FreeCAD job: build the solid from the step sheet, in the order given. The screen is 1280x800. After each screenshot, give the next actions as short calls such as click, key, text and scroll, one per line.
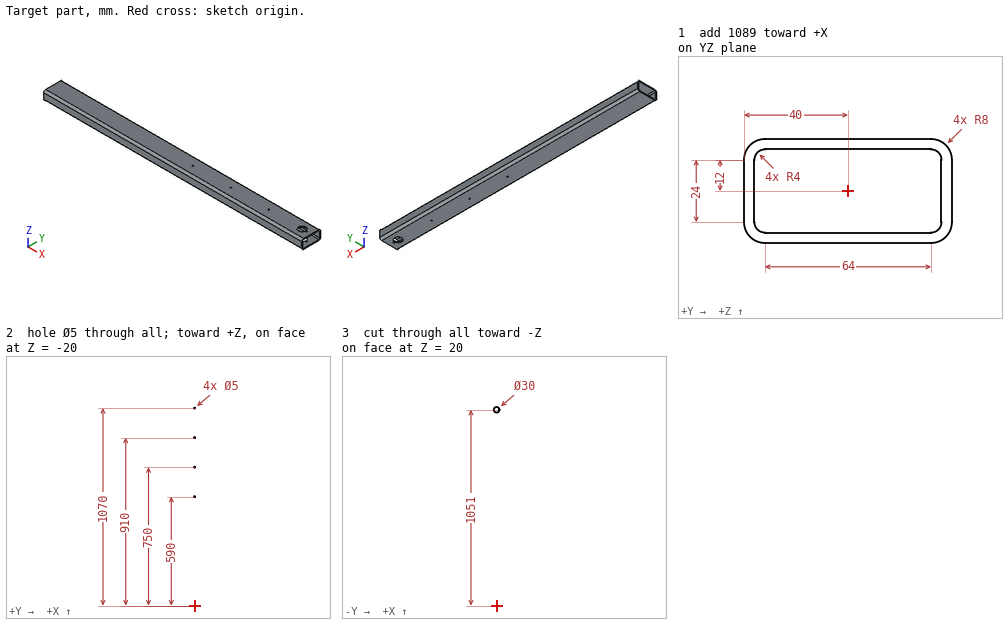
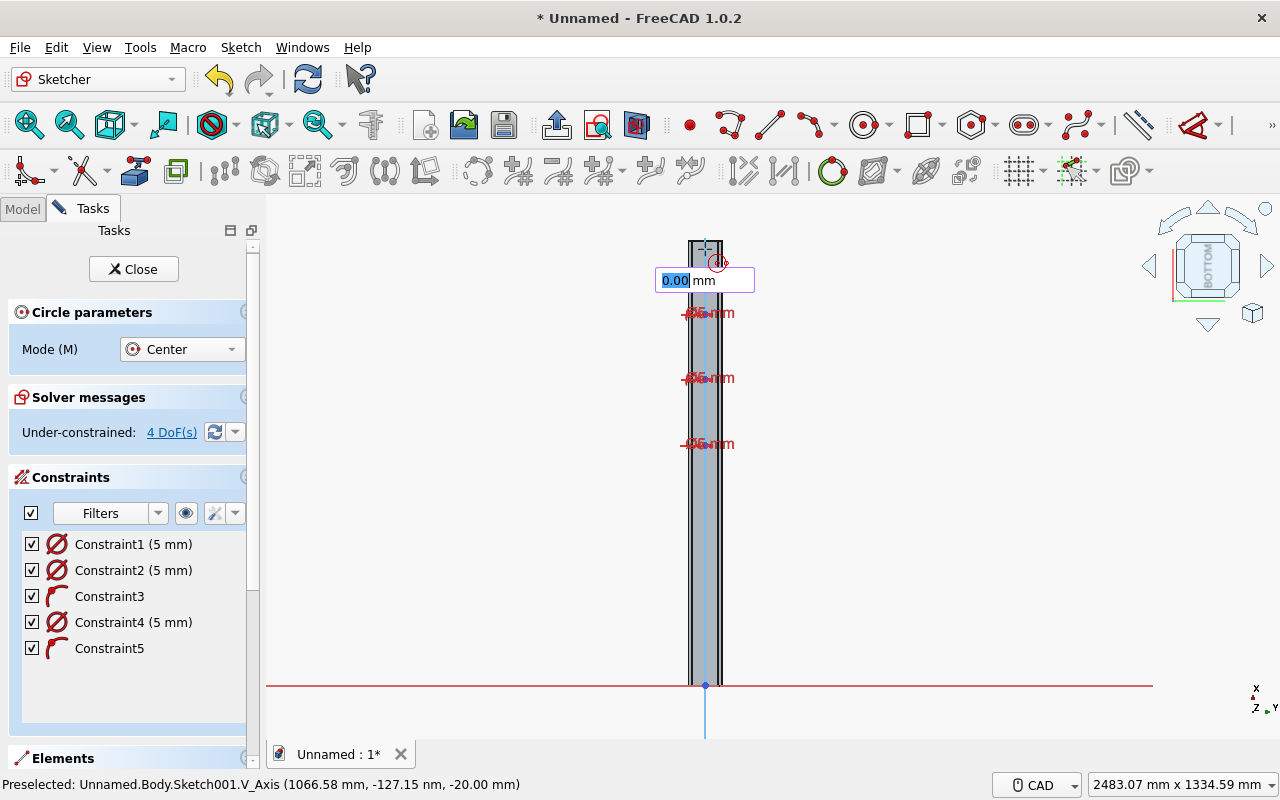
scroll(706, 248, up, 15)
move(703, 251)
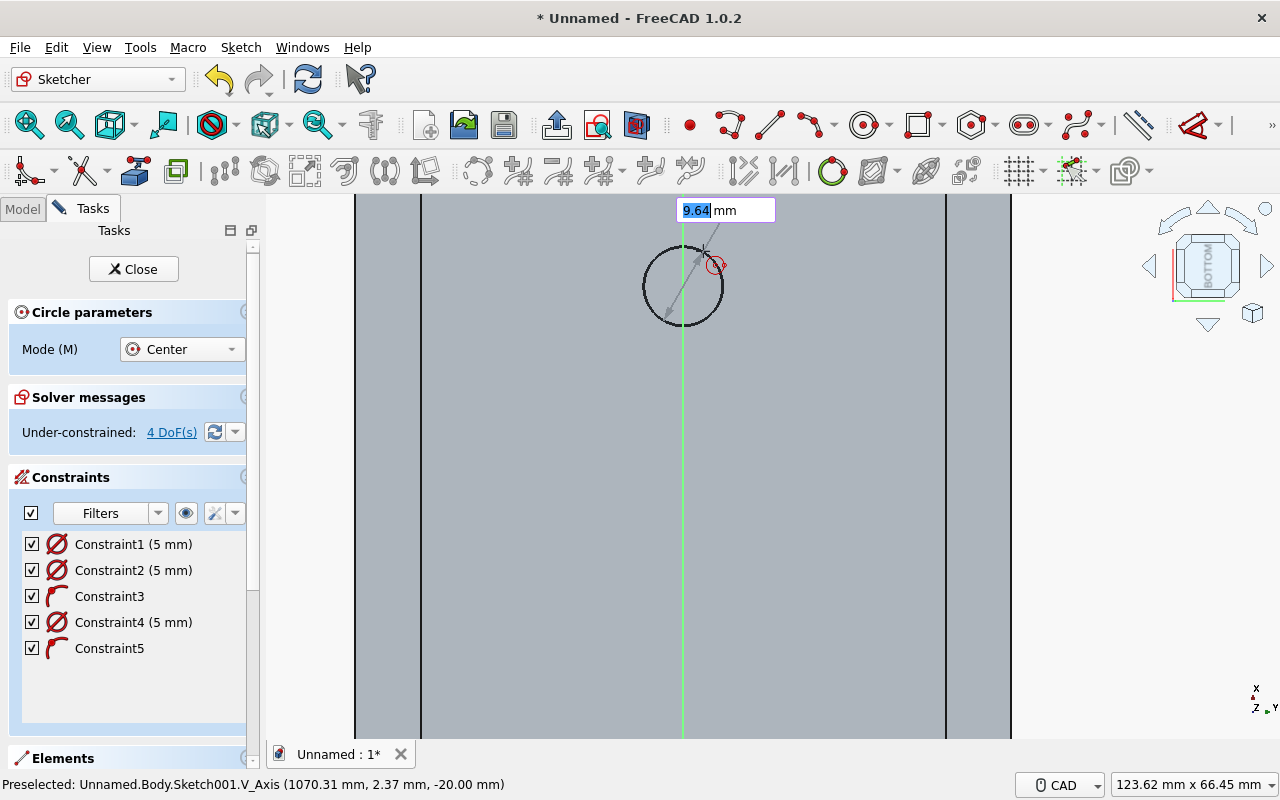
text(5)
key(Return)
key(Escape)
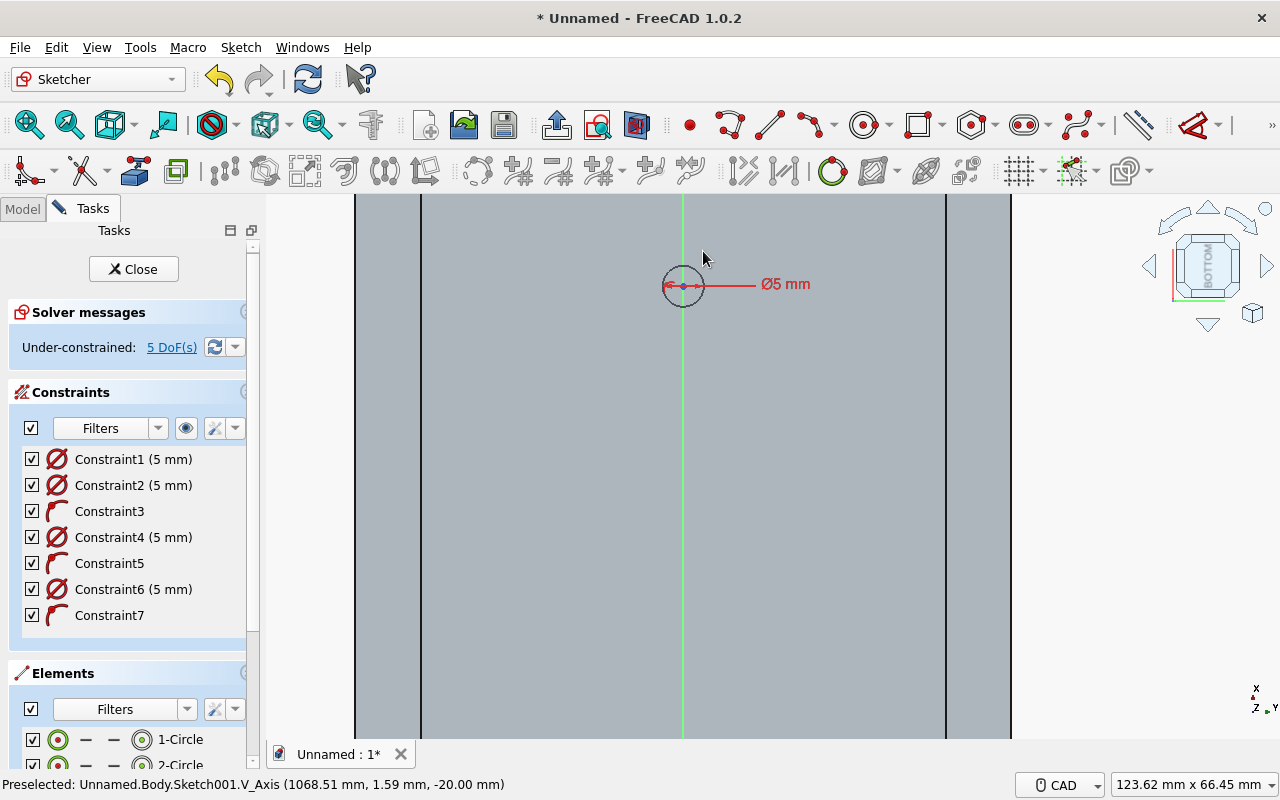
scroll(706, 248, down, 15)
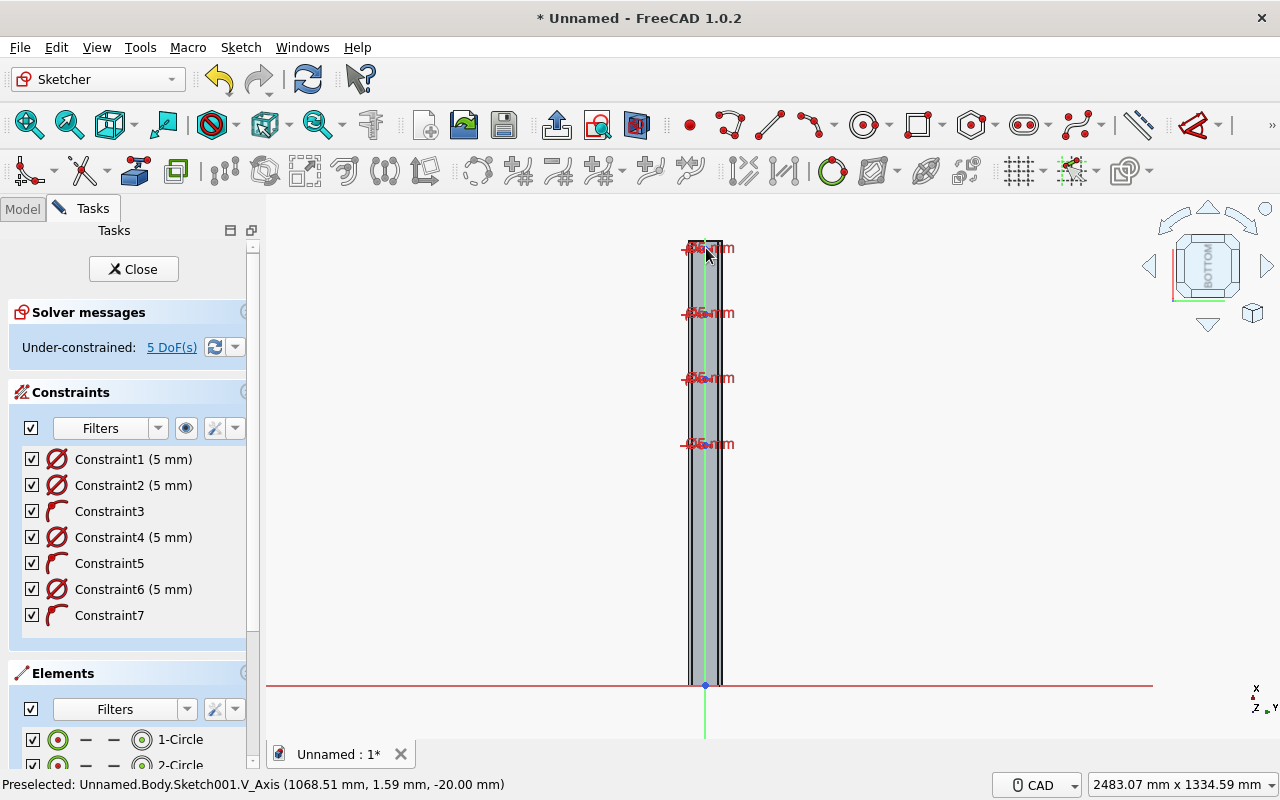
click(705, 446)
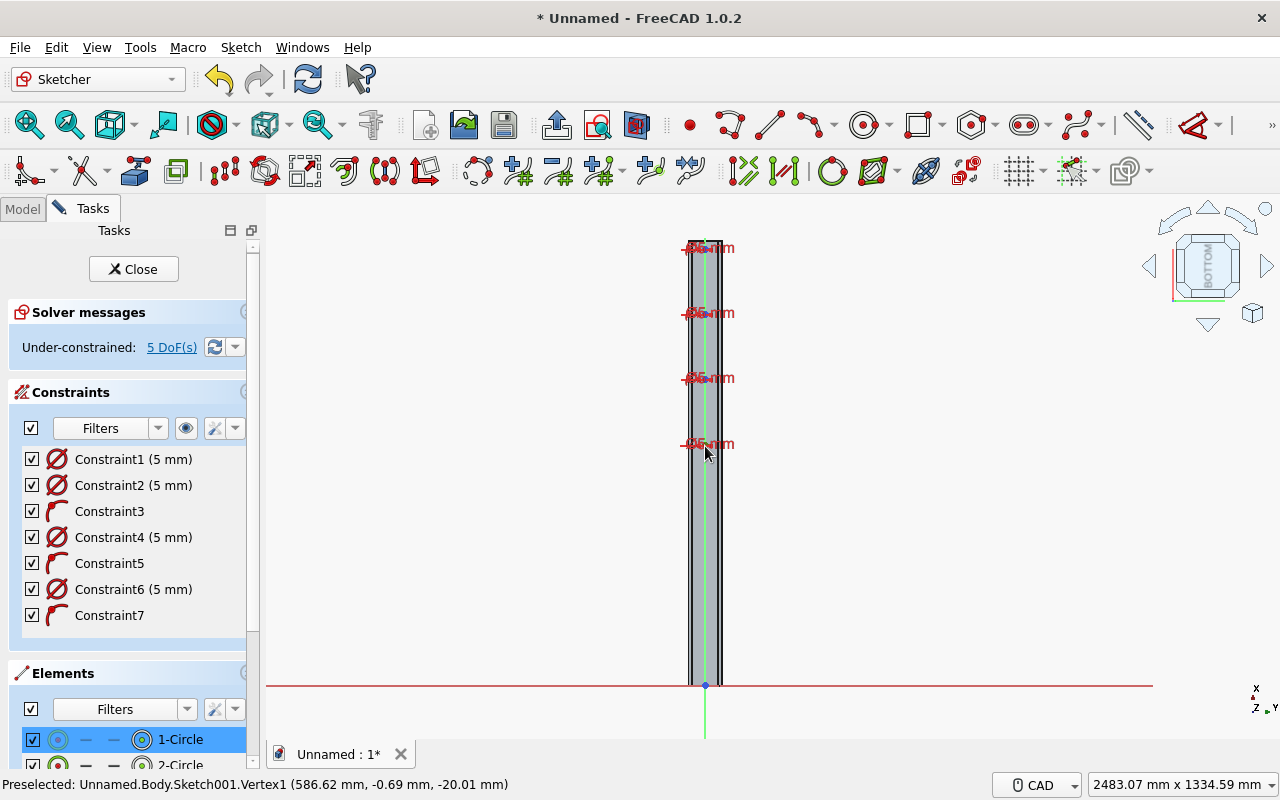
click(705, 641)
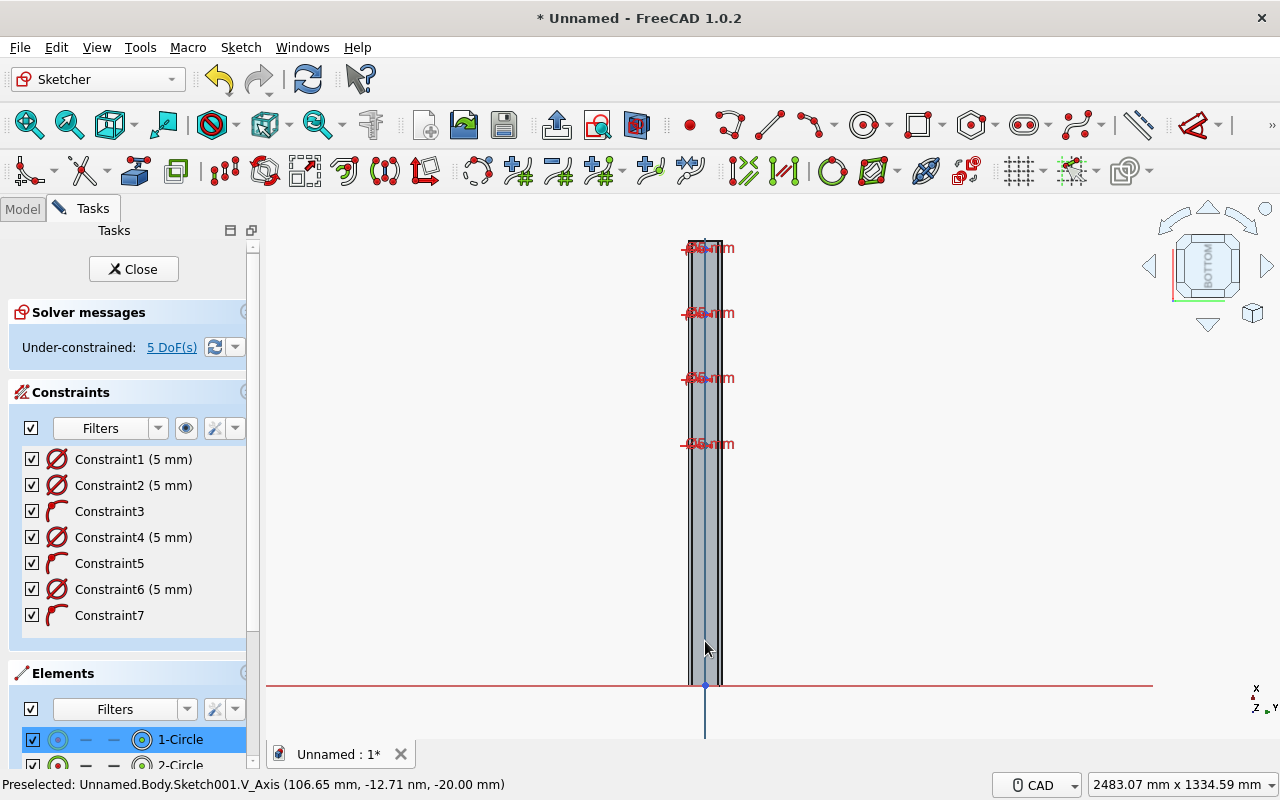
key(c)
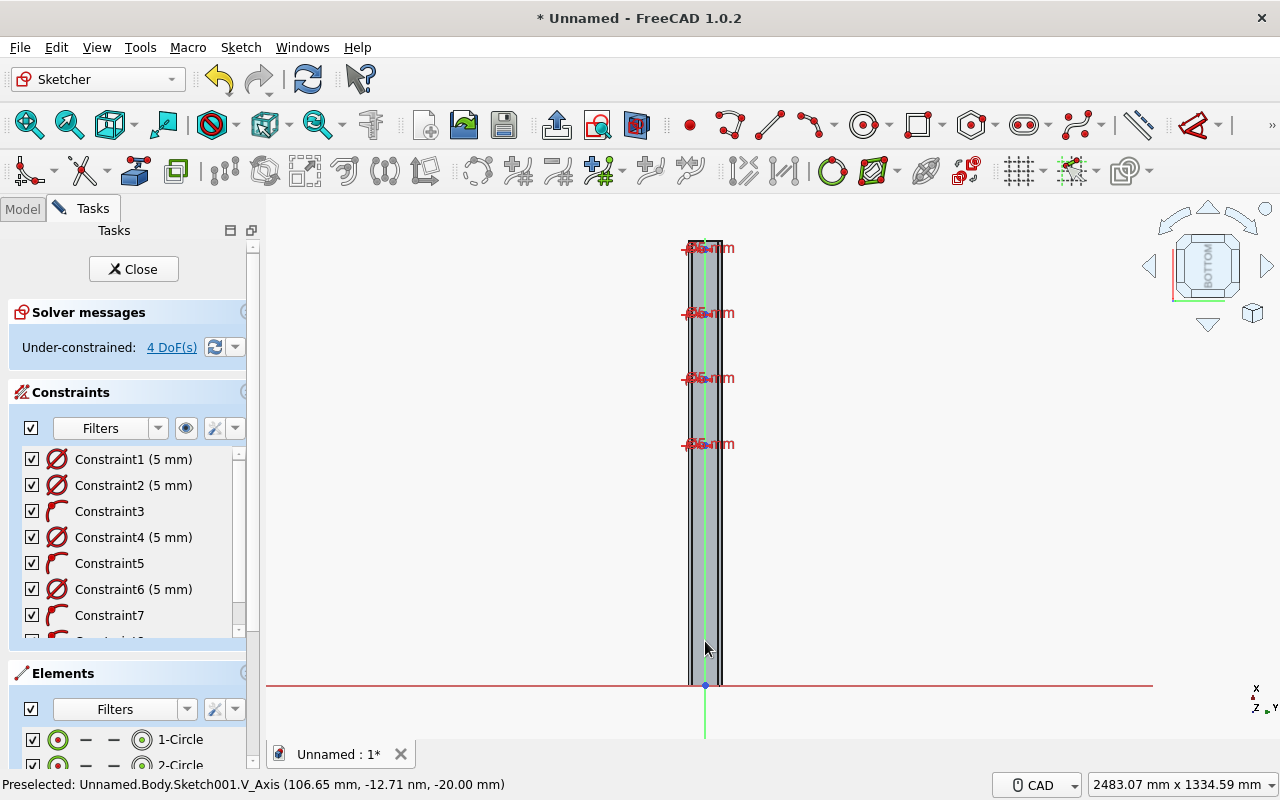
click(1194, 126)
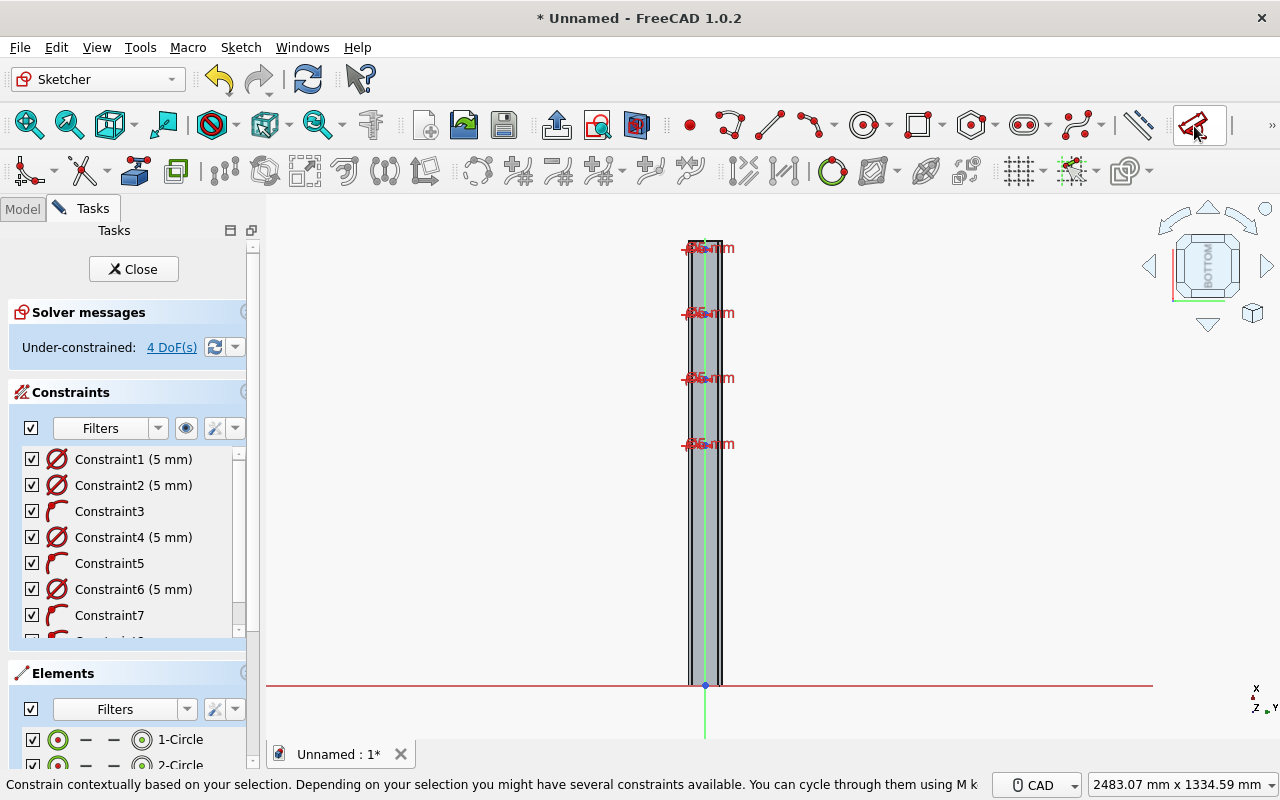
click(705, 446)
click(739, 566)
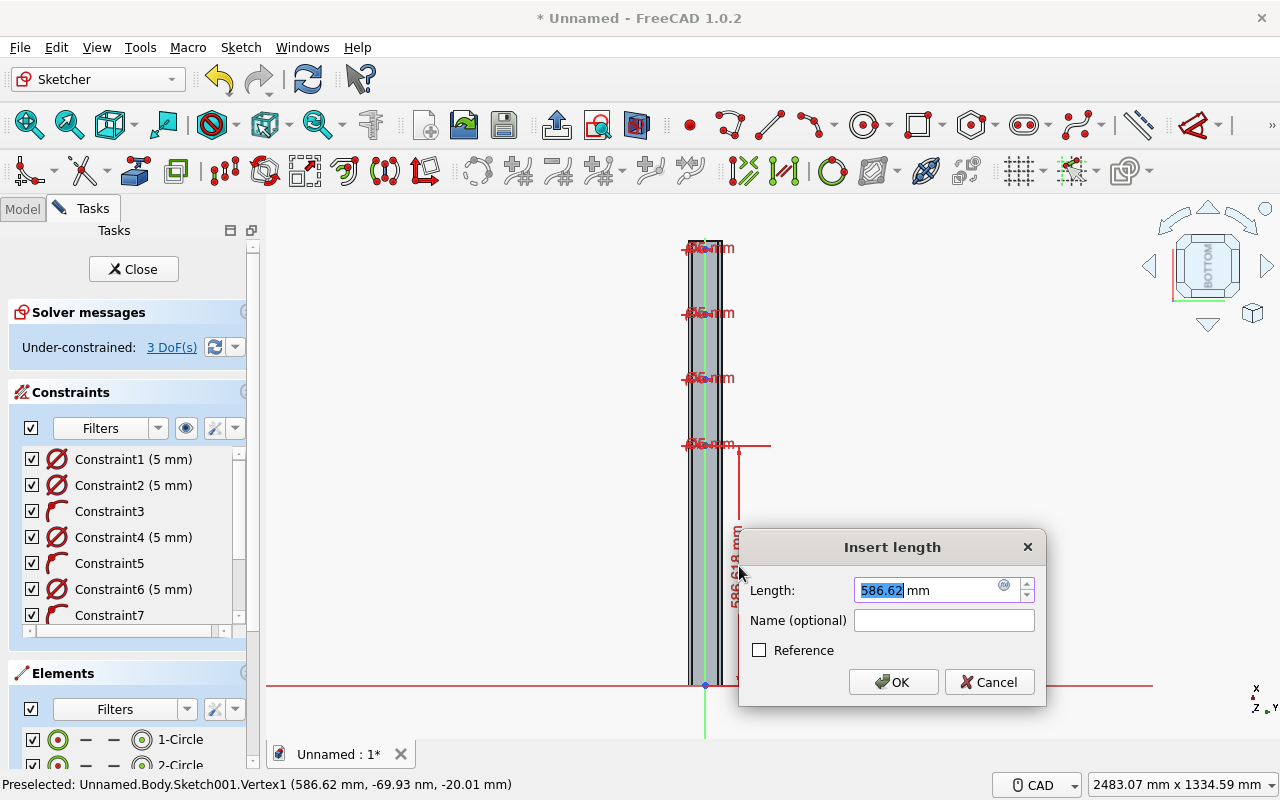
text(590)
key(Return)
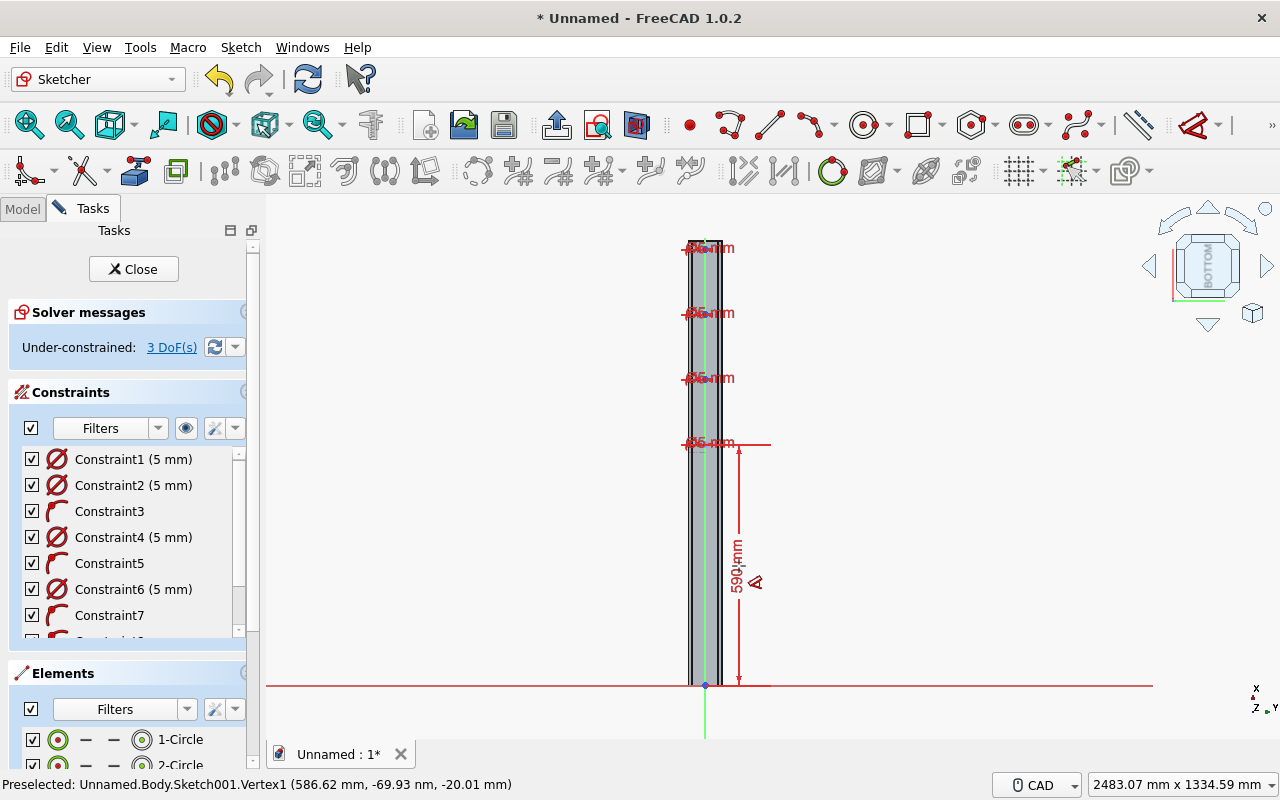
click(705, 380)
click(739, 533)